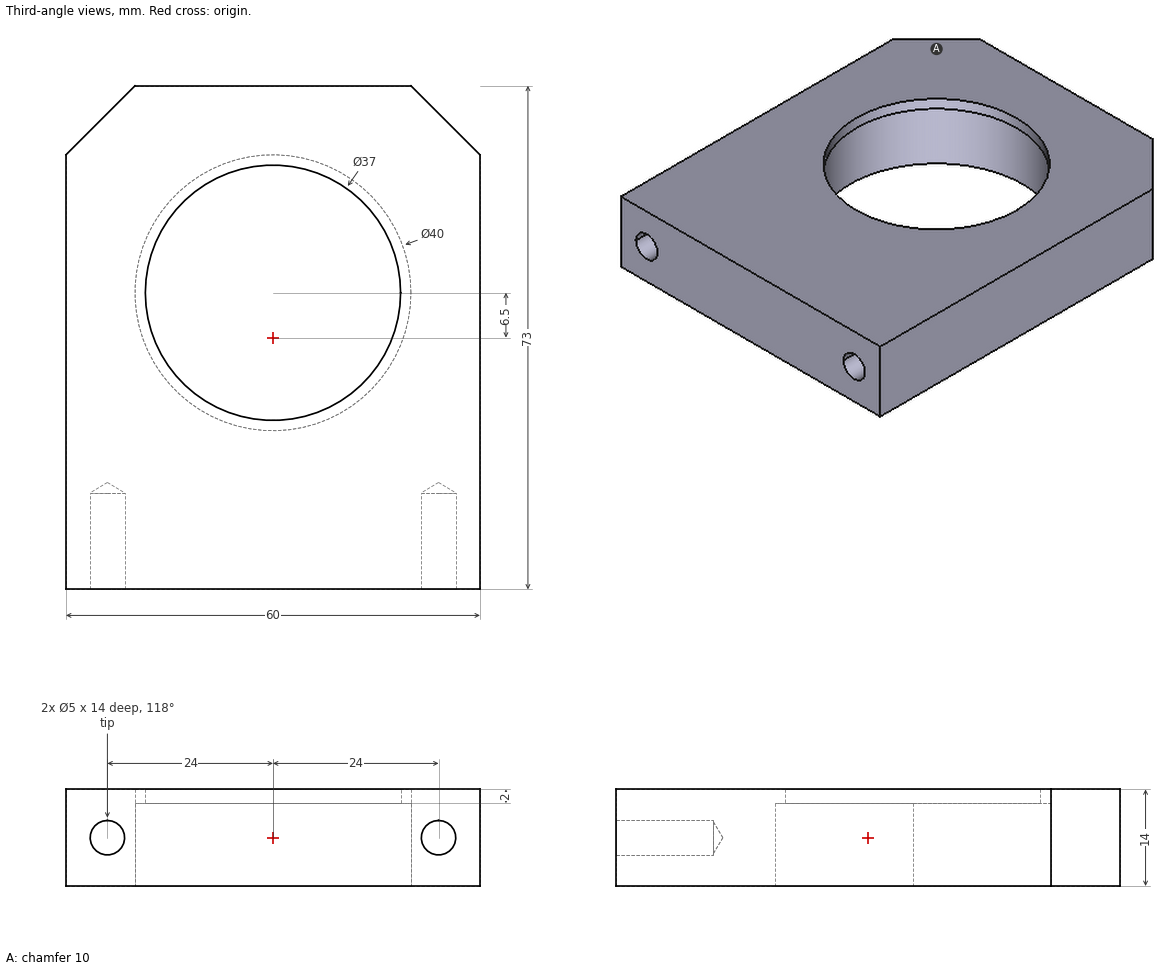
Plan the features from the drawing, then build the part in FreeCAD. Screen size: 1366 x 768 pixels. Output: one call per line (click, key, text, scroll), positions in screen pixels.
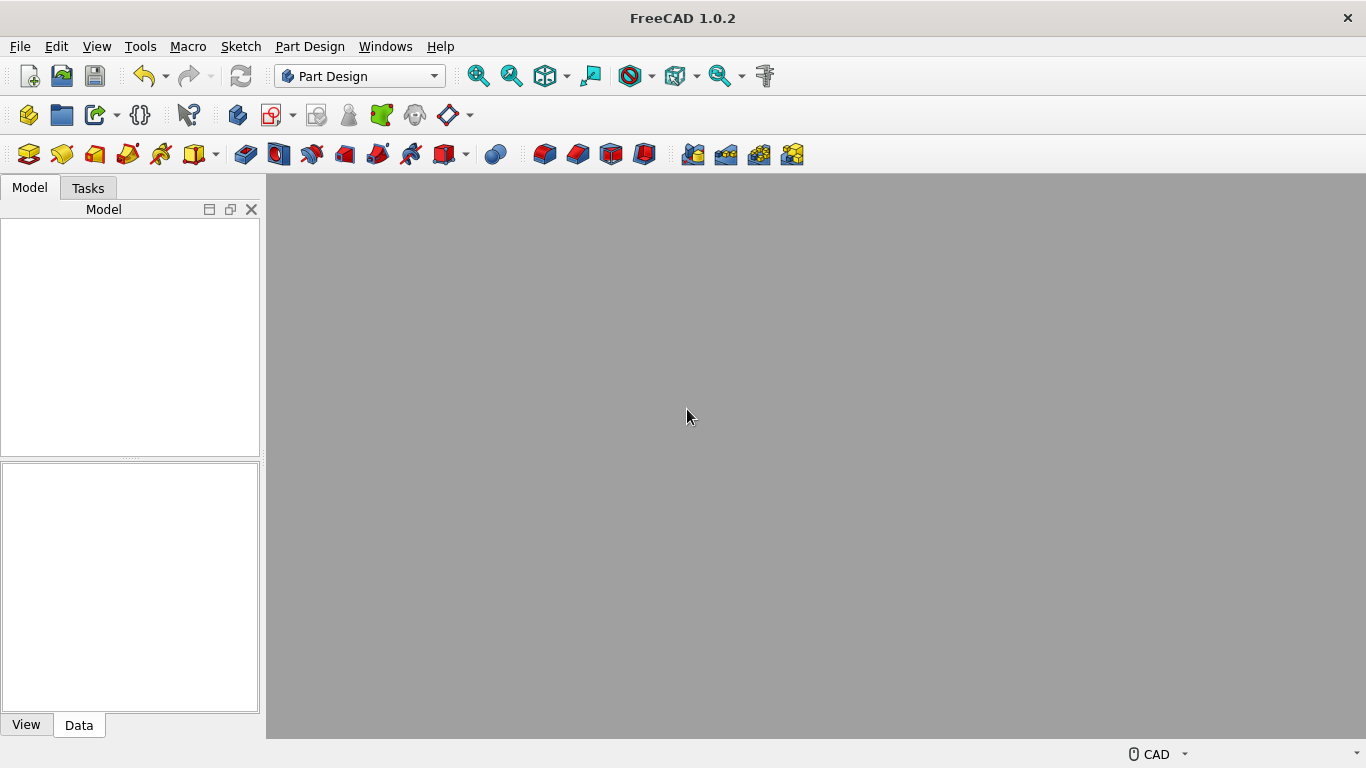
click(29, 76)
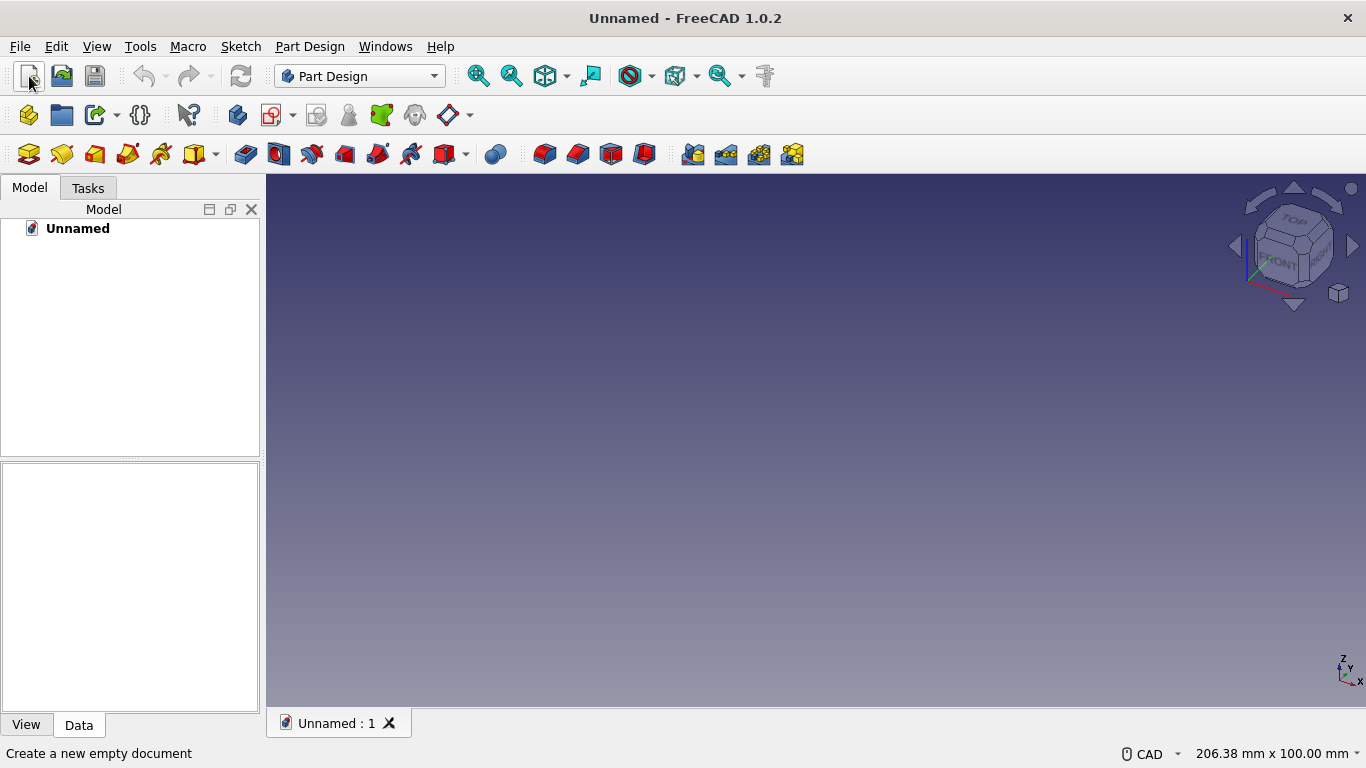
click(270, 116)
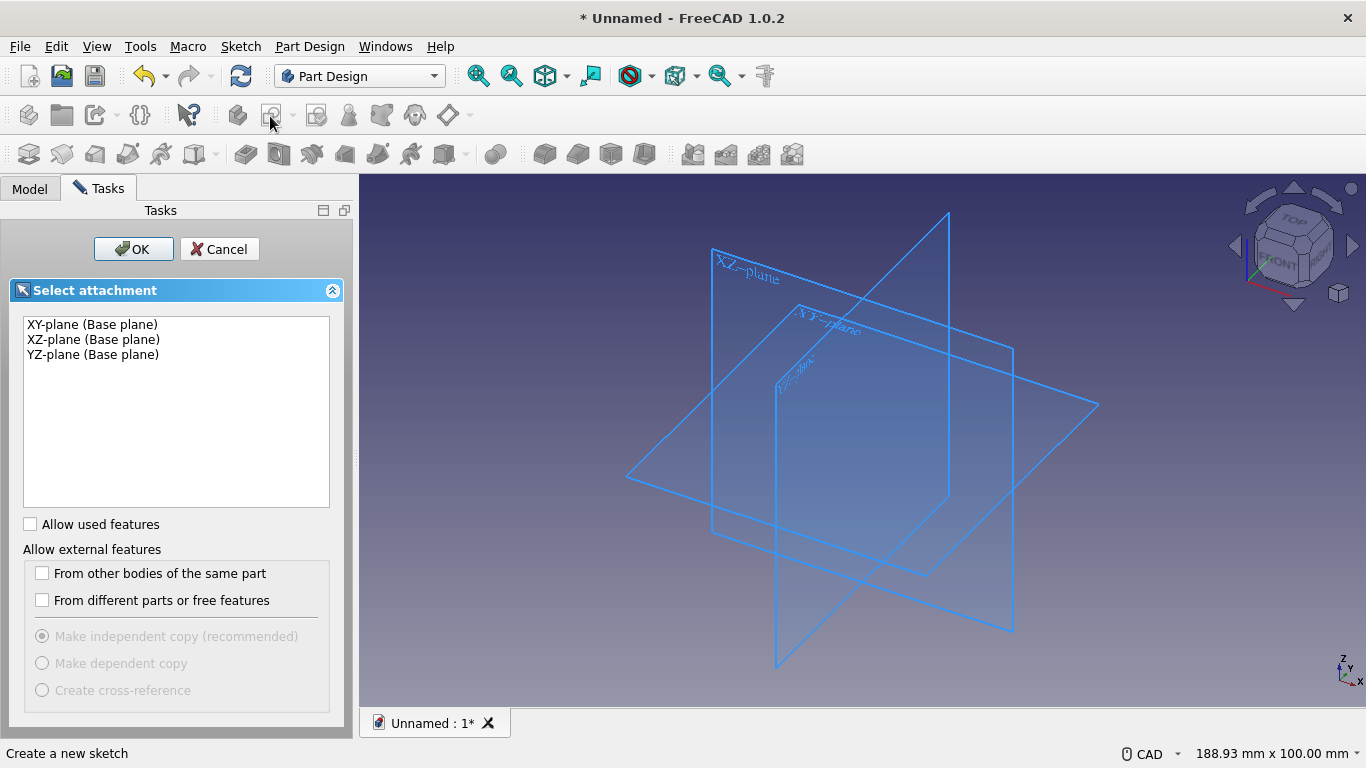
click(84, 324)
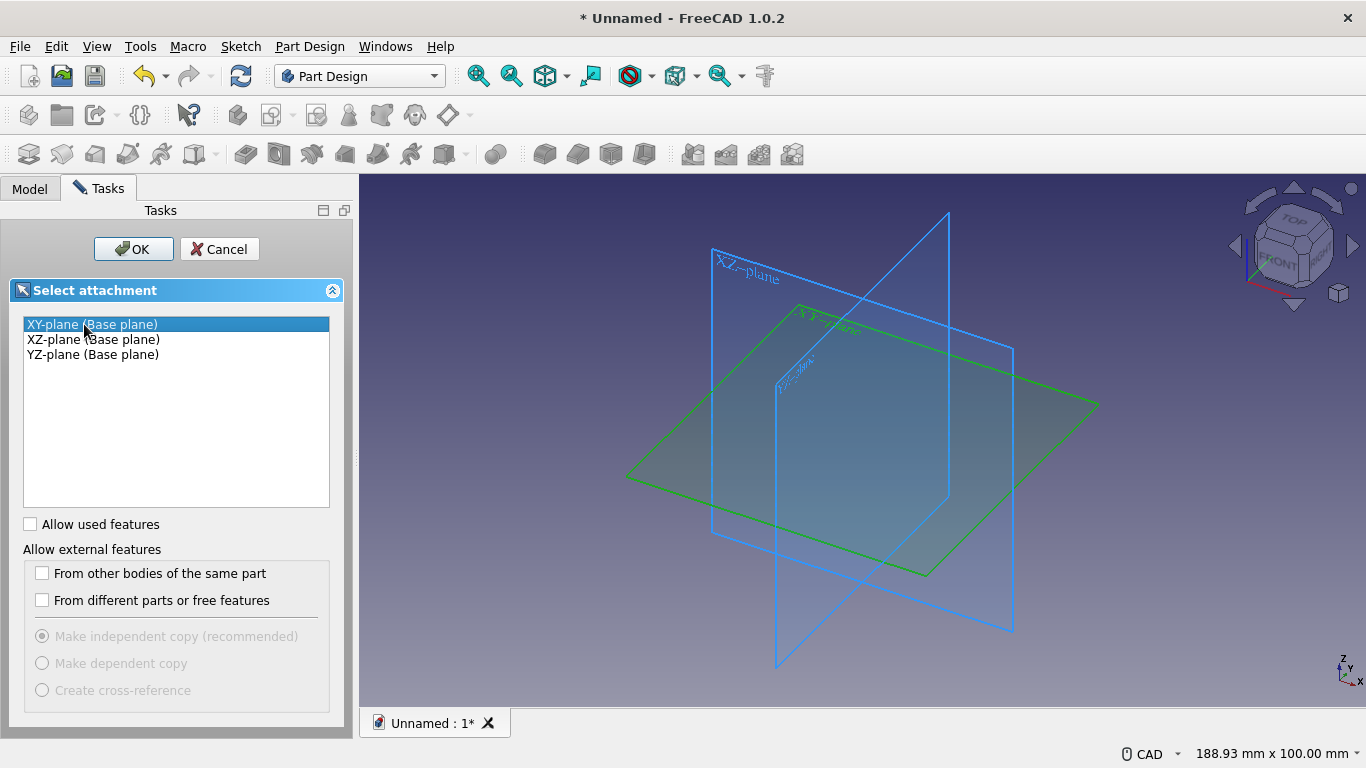
click(134, 249)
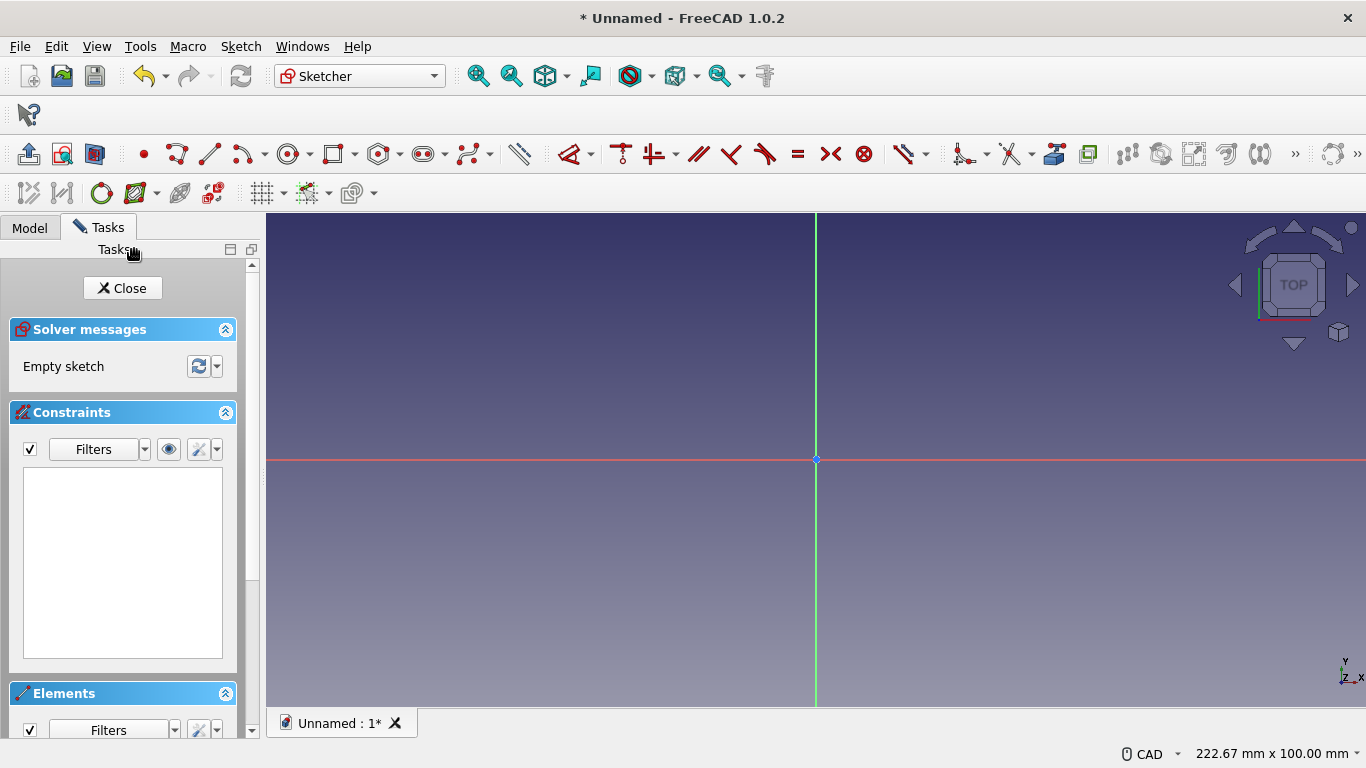
click(354, 154)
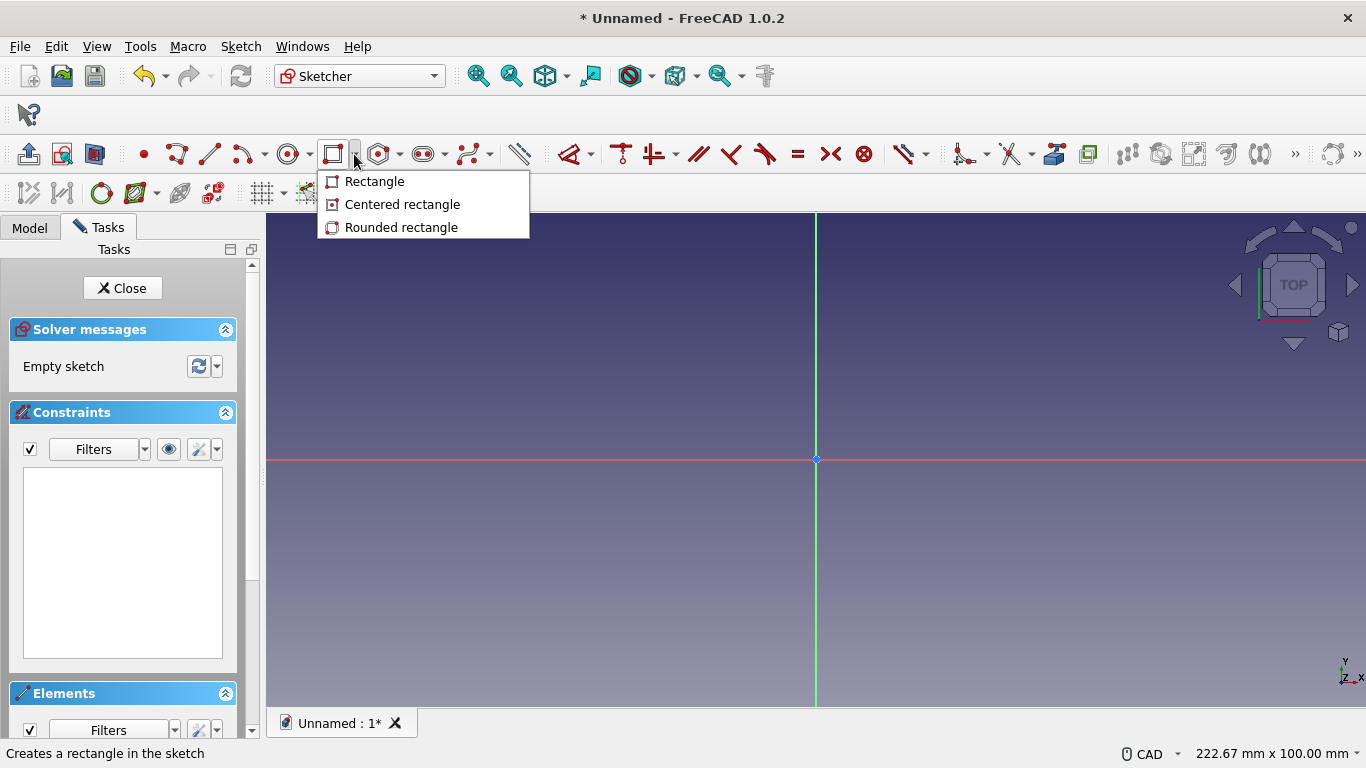
click(424, 204)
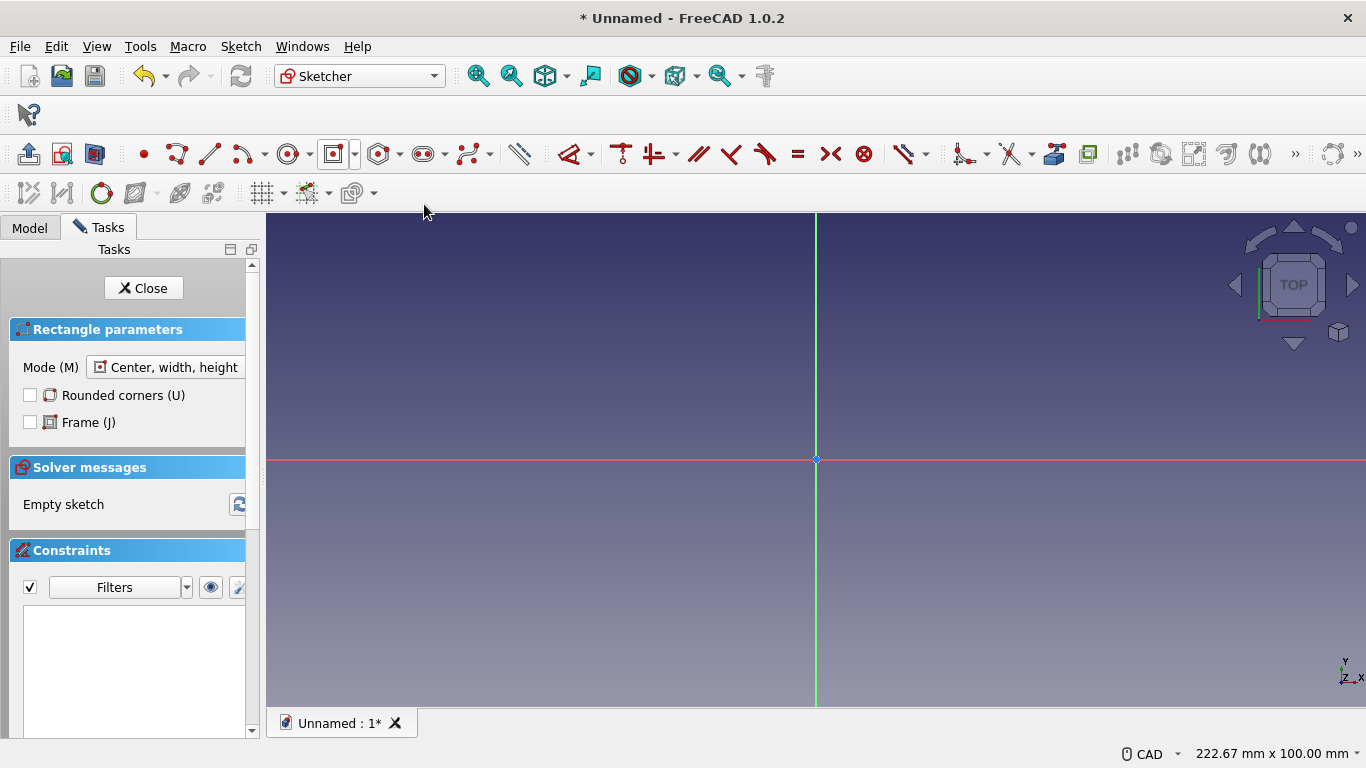
click(816, 460)
move(964, 280)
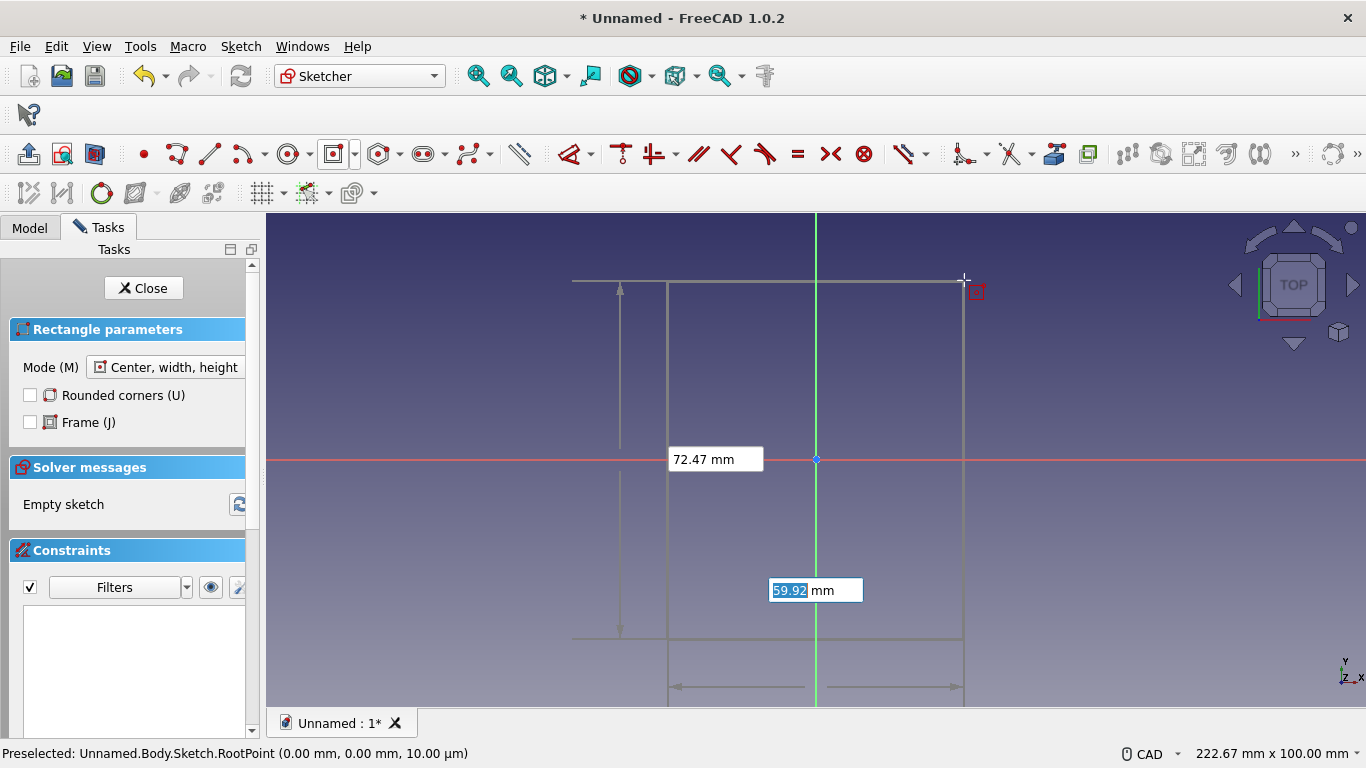
text(60)
key(Tab)
text(73)
key(Return)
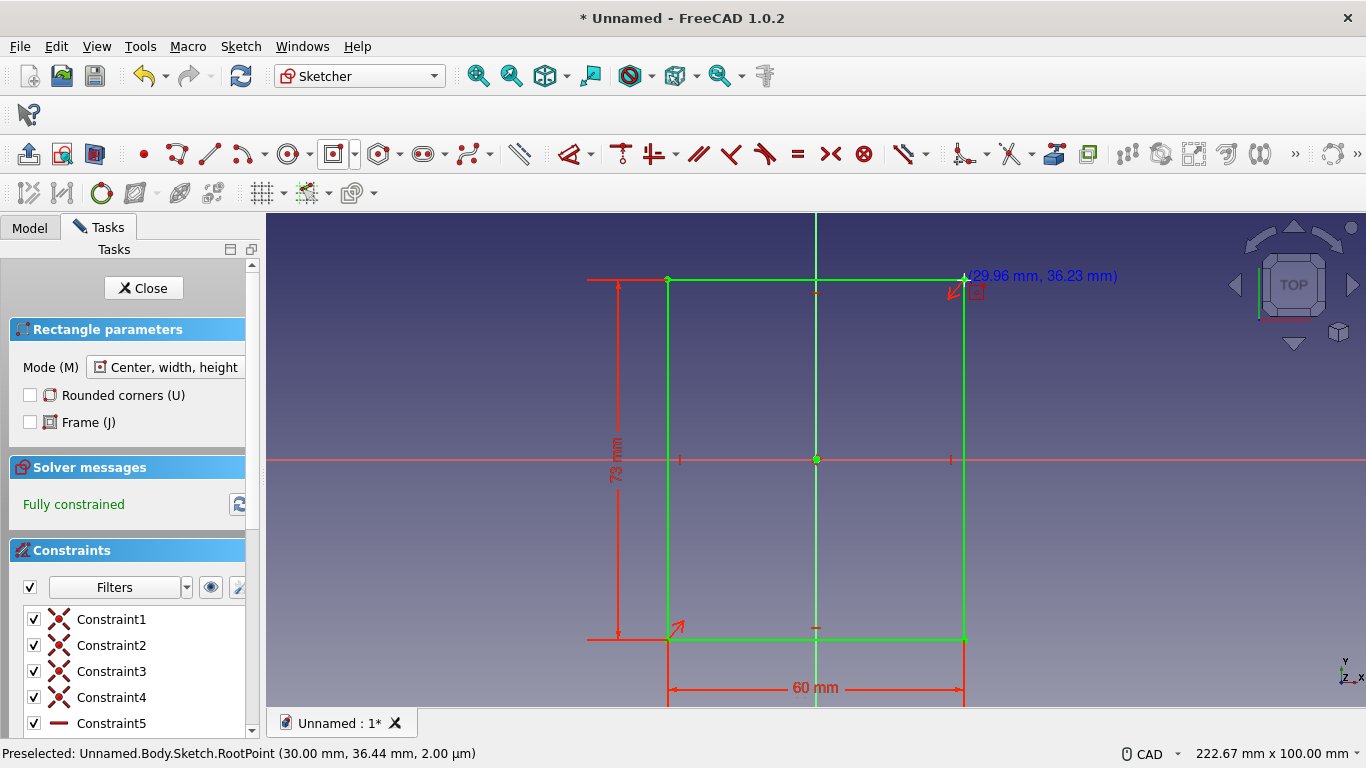
click(288, 154)